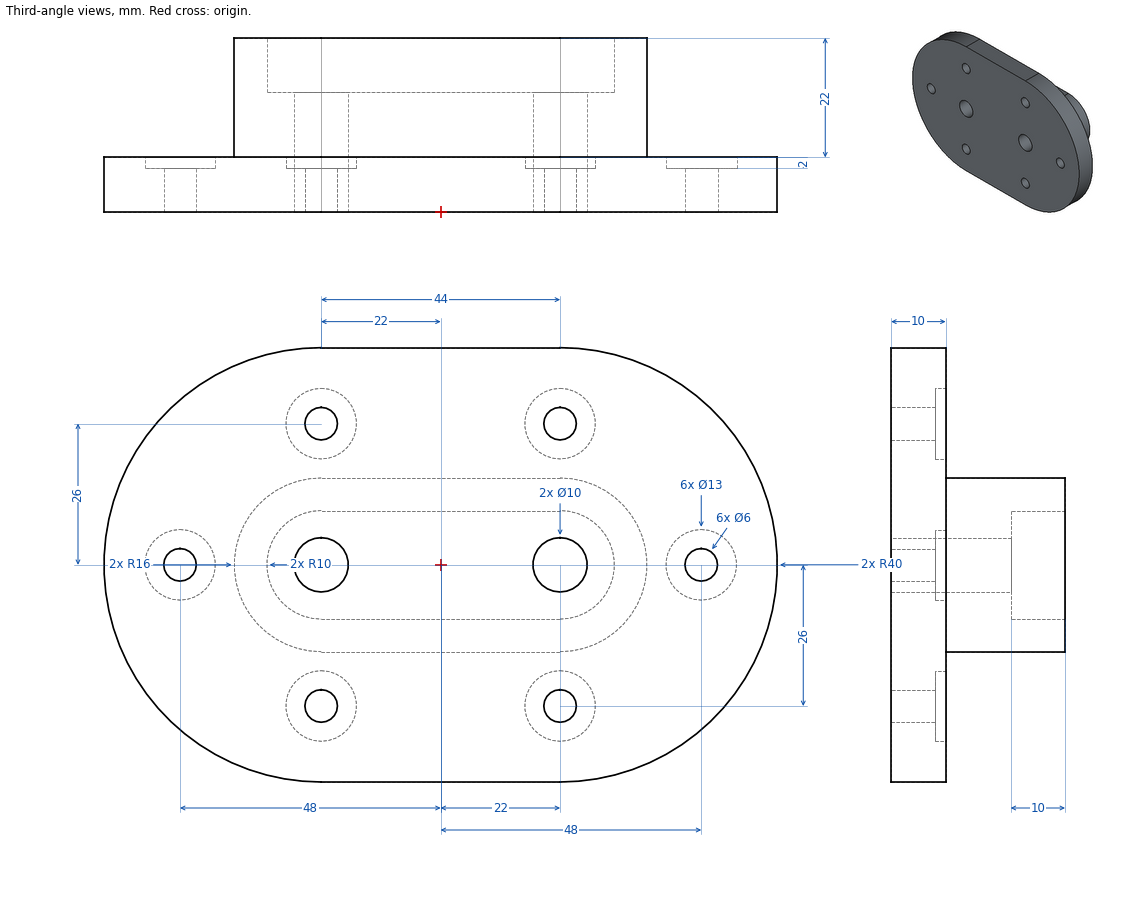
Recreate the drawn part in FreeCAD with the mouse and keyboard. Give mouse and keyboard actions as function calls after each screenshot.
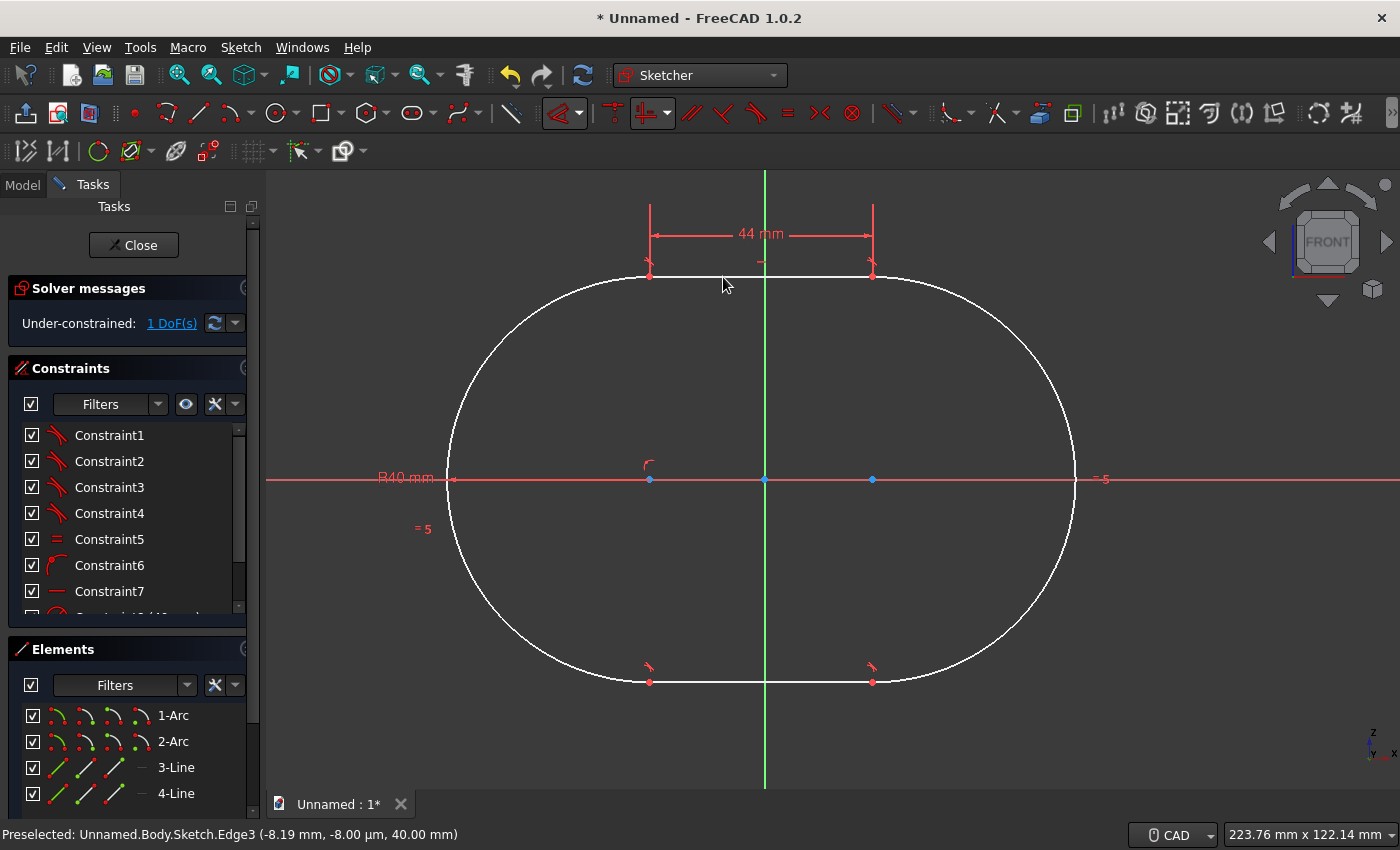
click(650, 277)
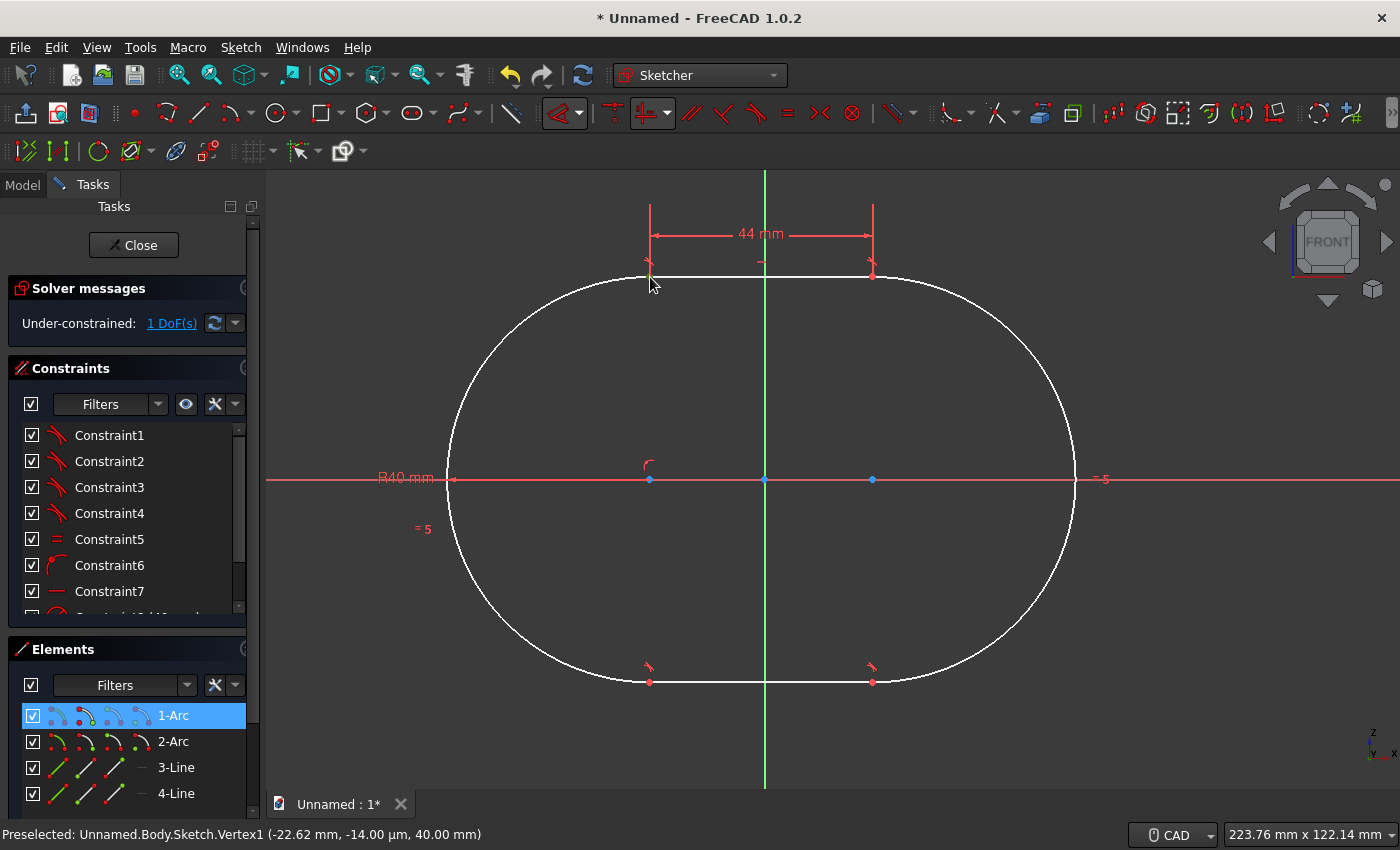
click(582, 114)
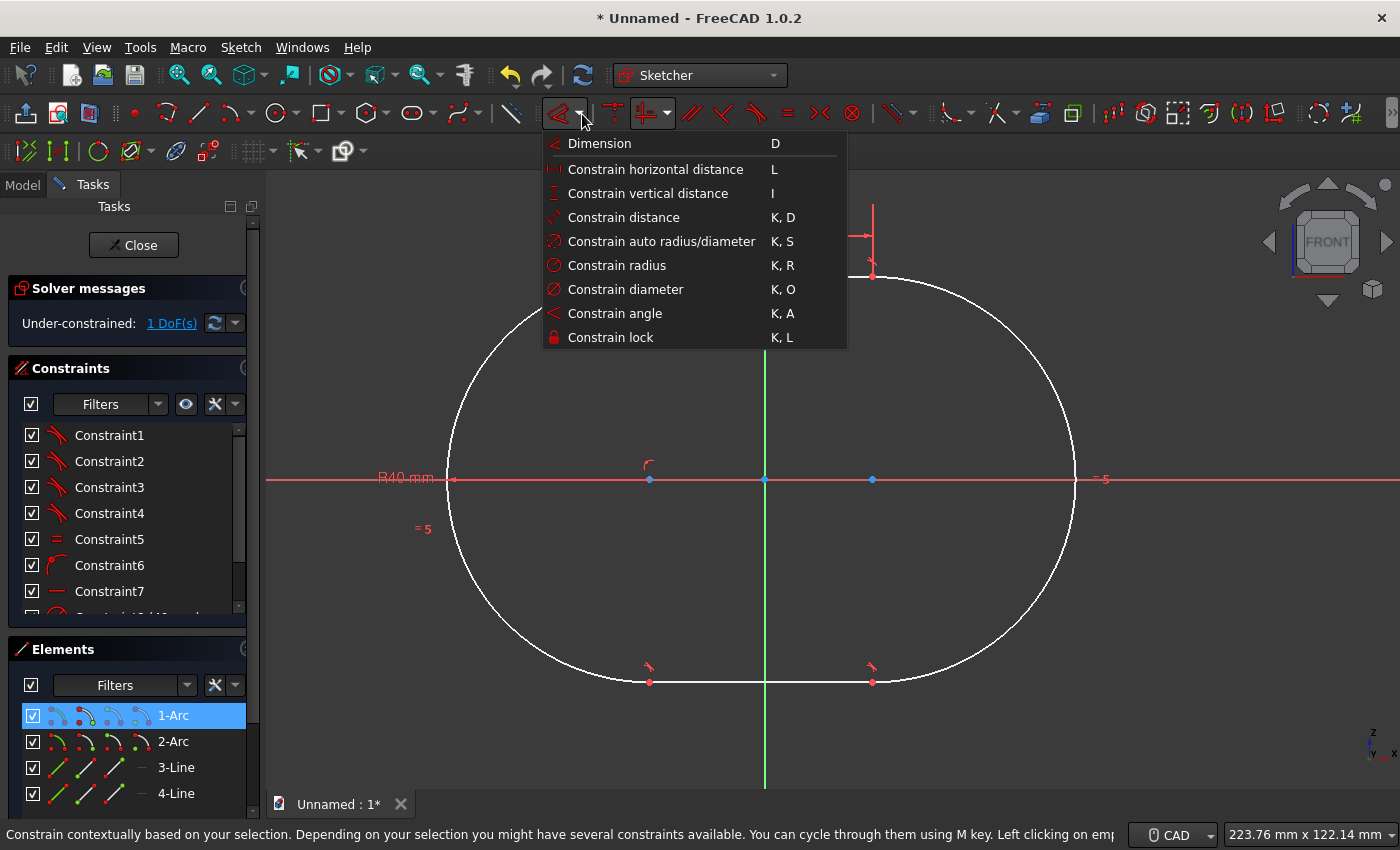
click(695, 169)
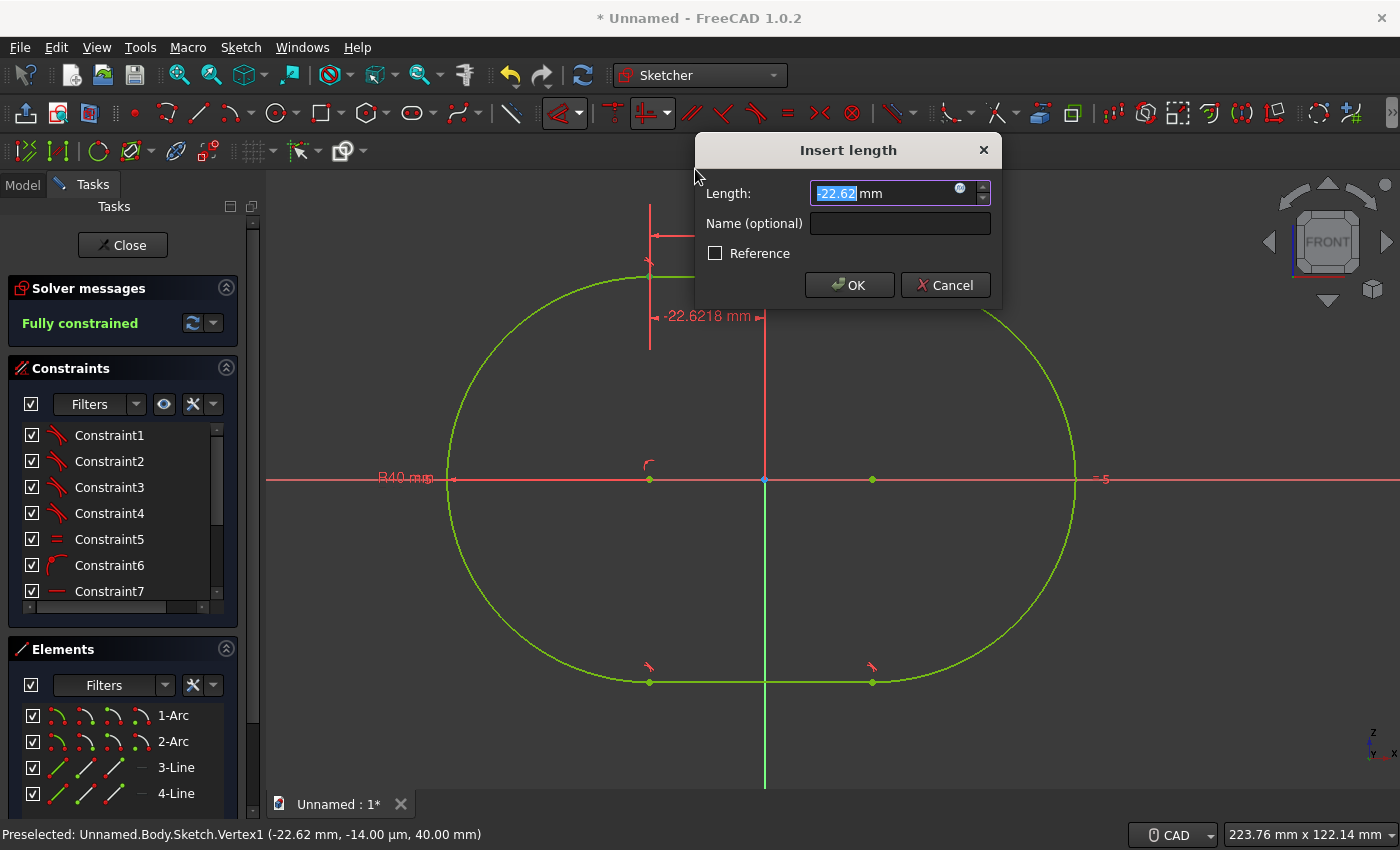
text(-22)
key(Return)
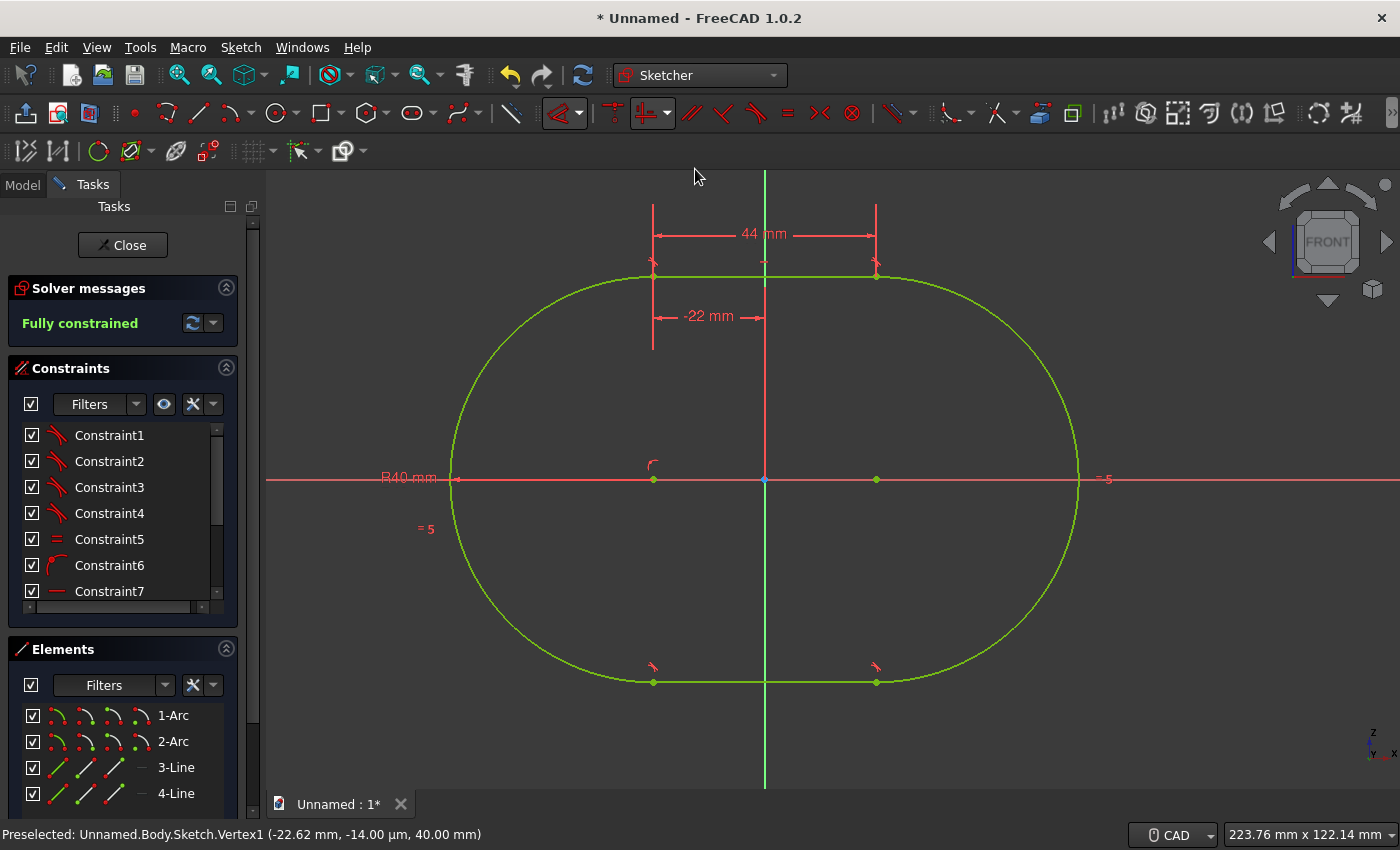
click(123, 245)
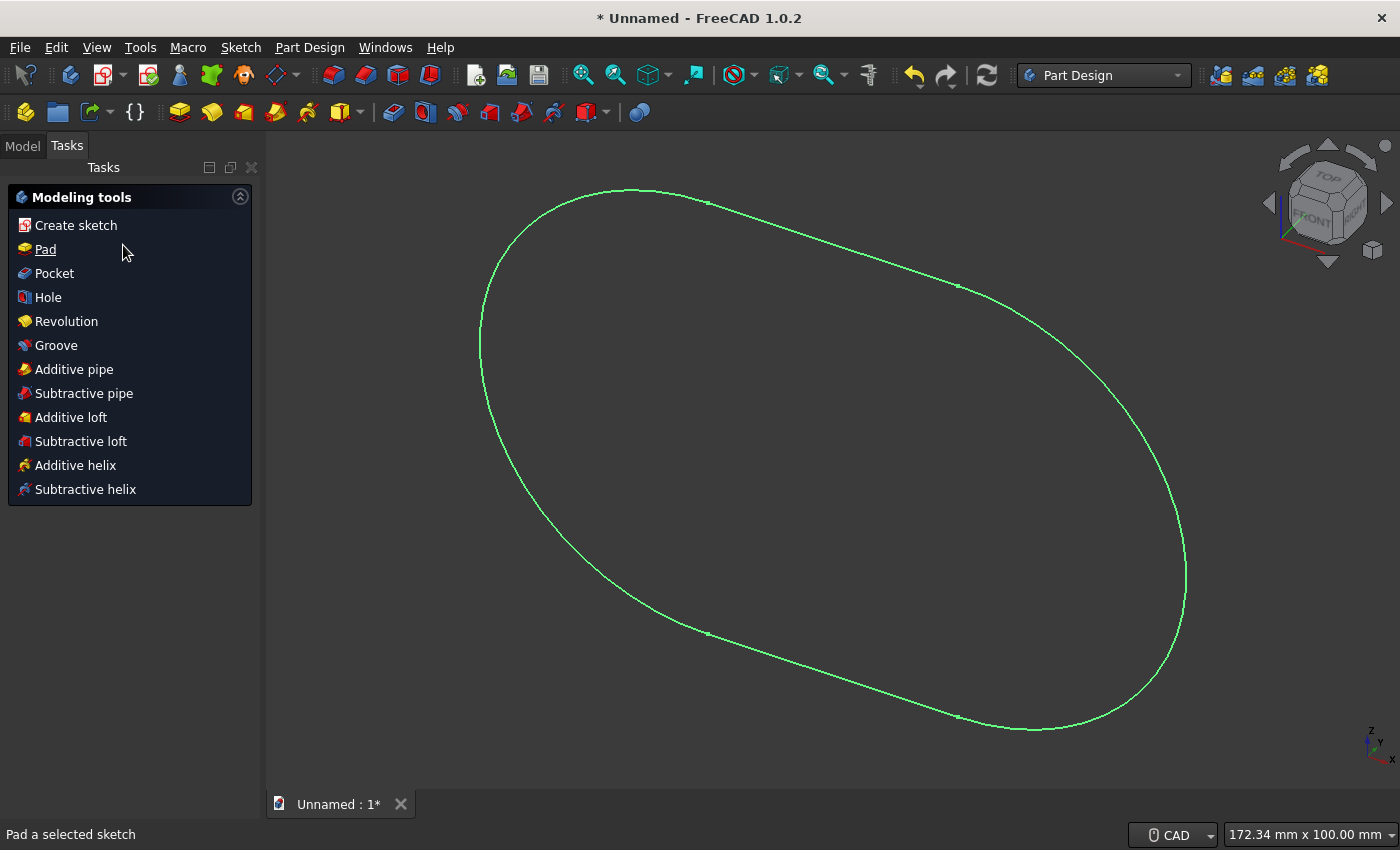
click(180, 112)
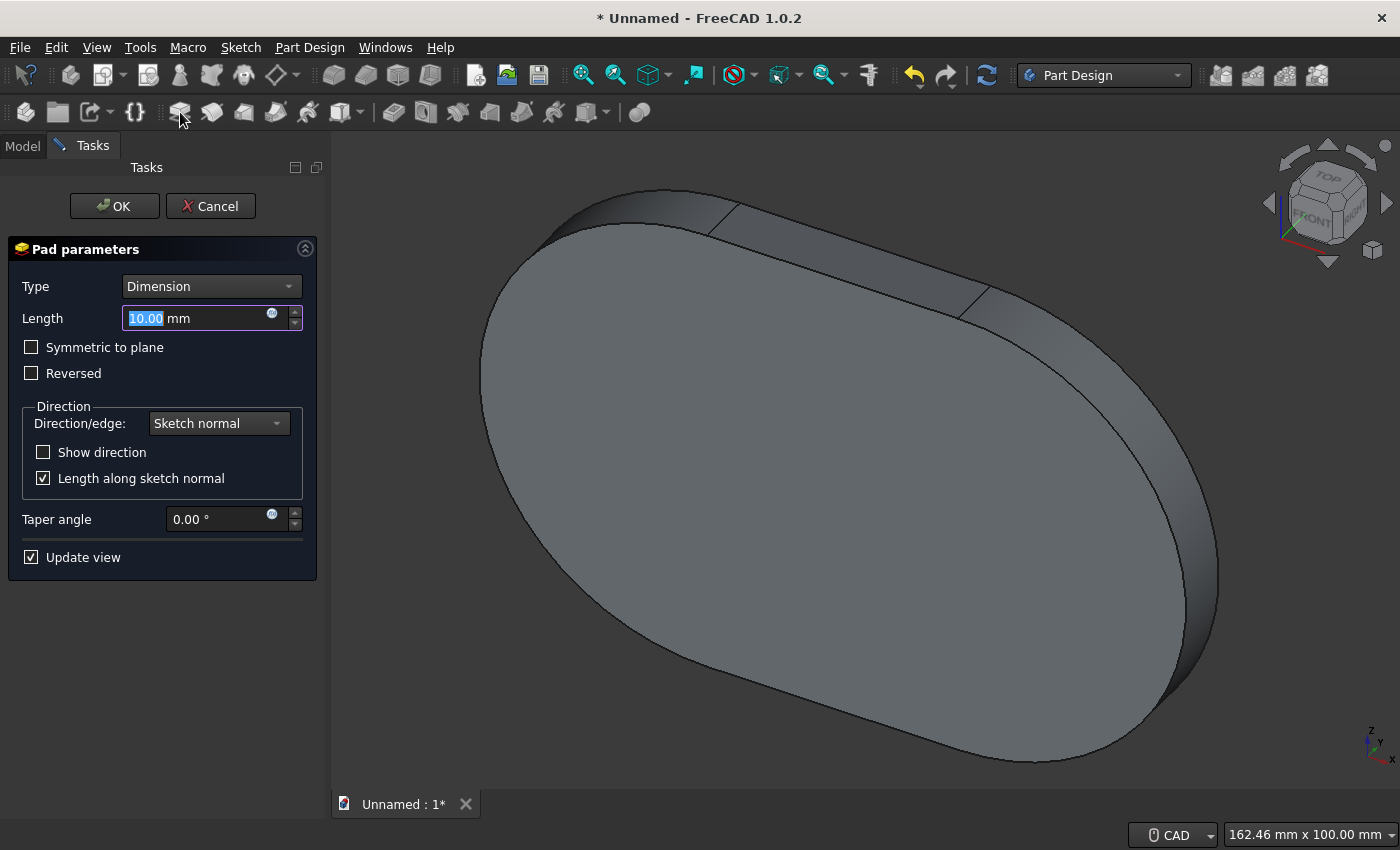
text(10)
key(Tab)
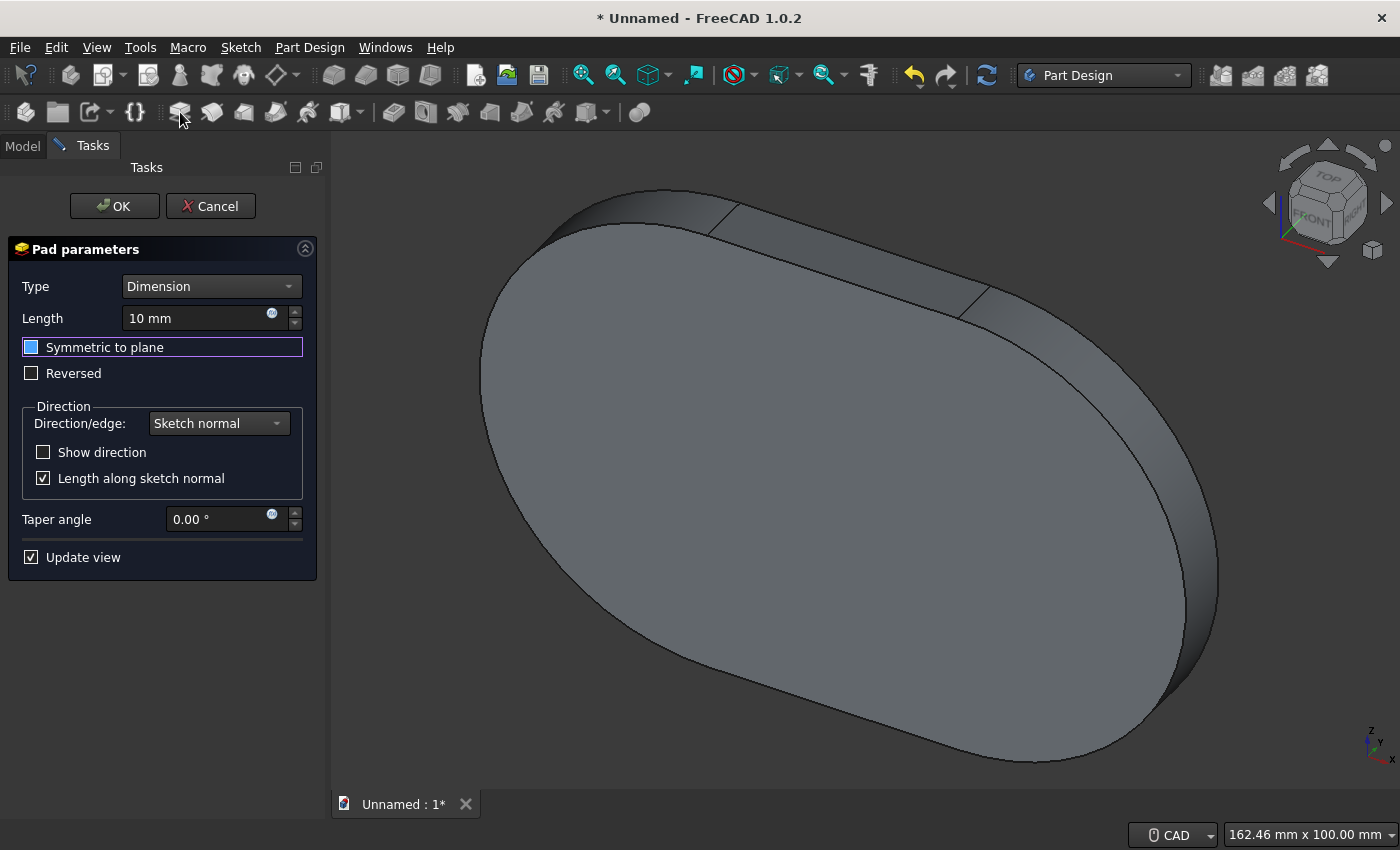
click(30, 373)